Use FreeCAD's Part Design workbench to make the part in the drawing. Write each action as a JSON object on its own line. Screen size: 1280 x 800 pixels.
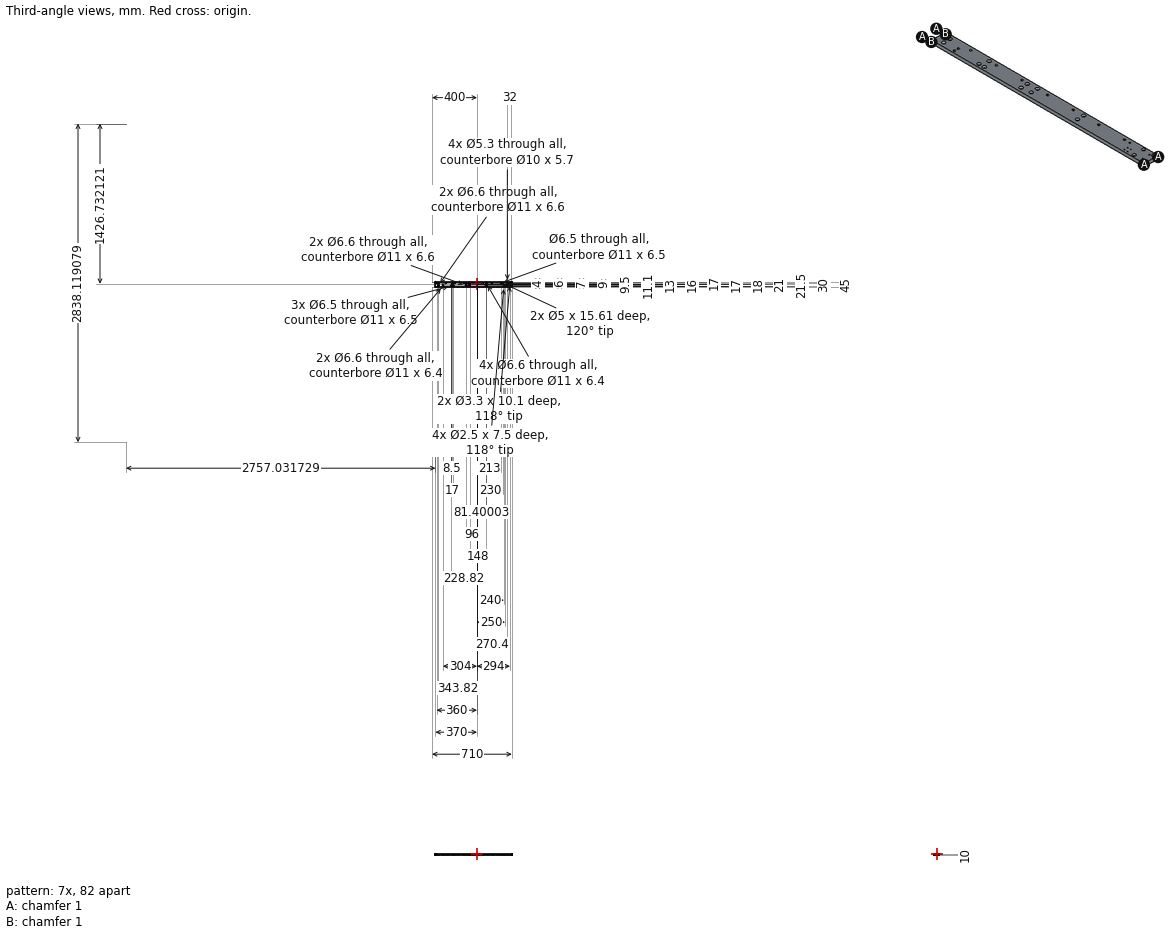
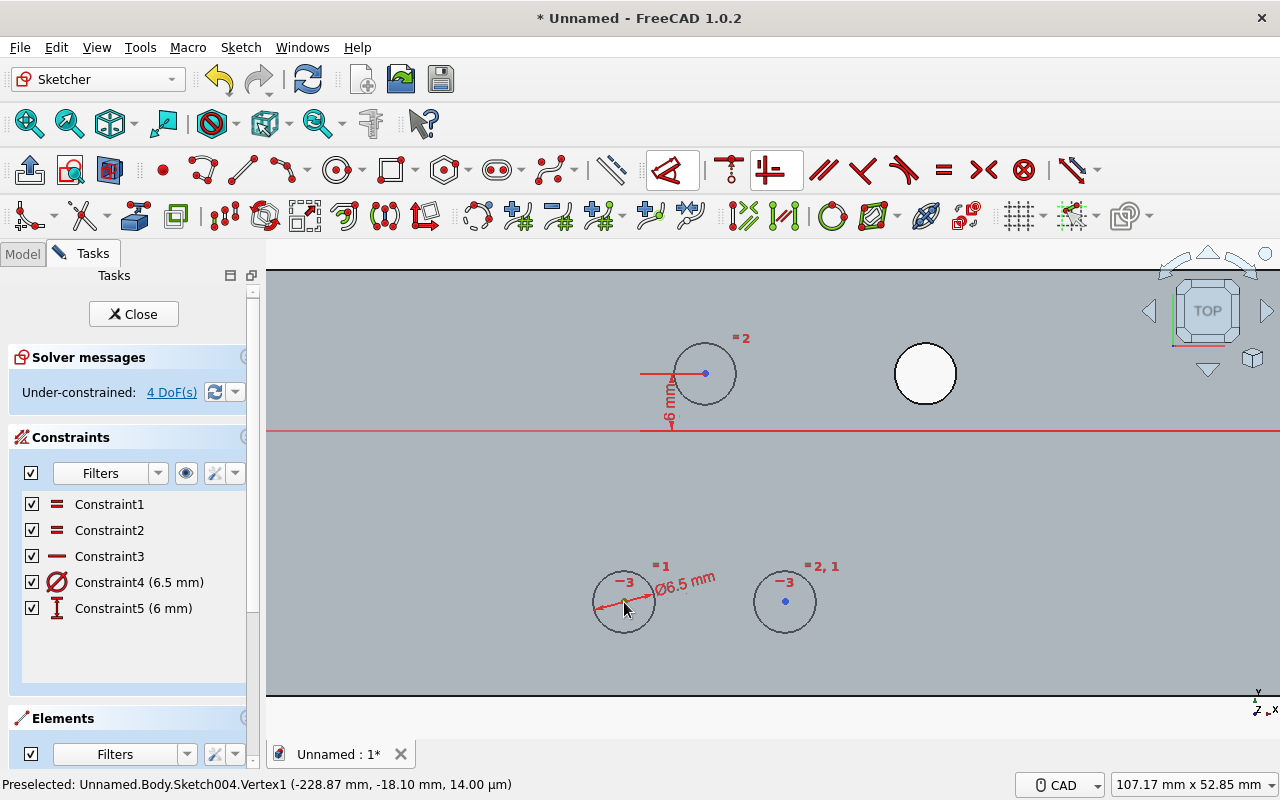
{"action": "left_click", "coordinate": [694, 170]}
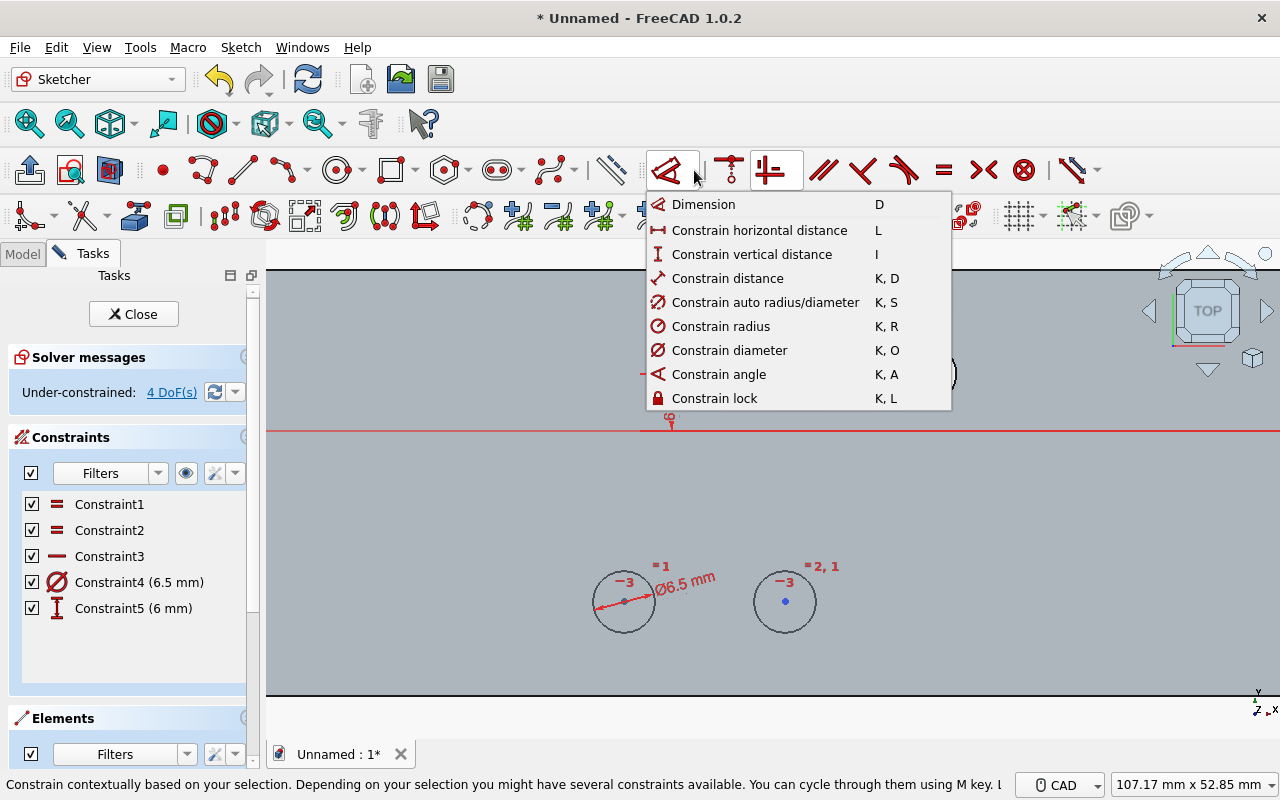
{"action": "left_click", "coordinate": [799, 254]}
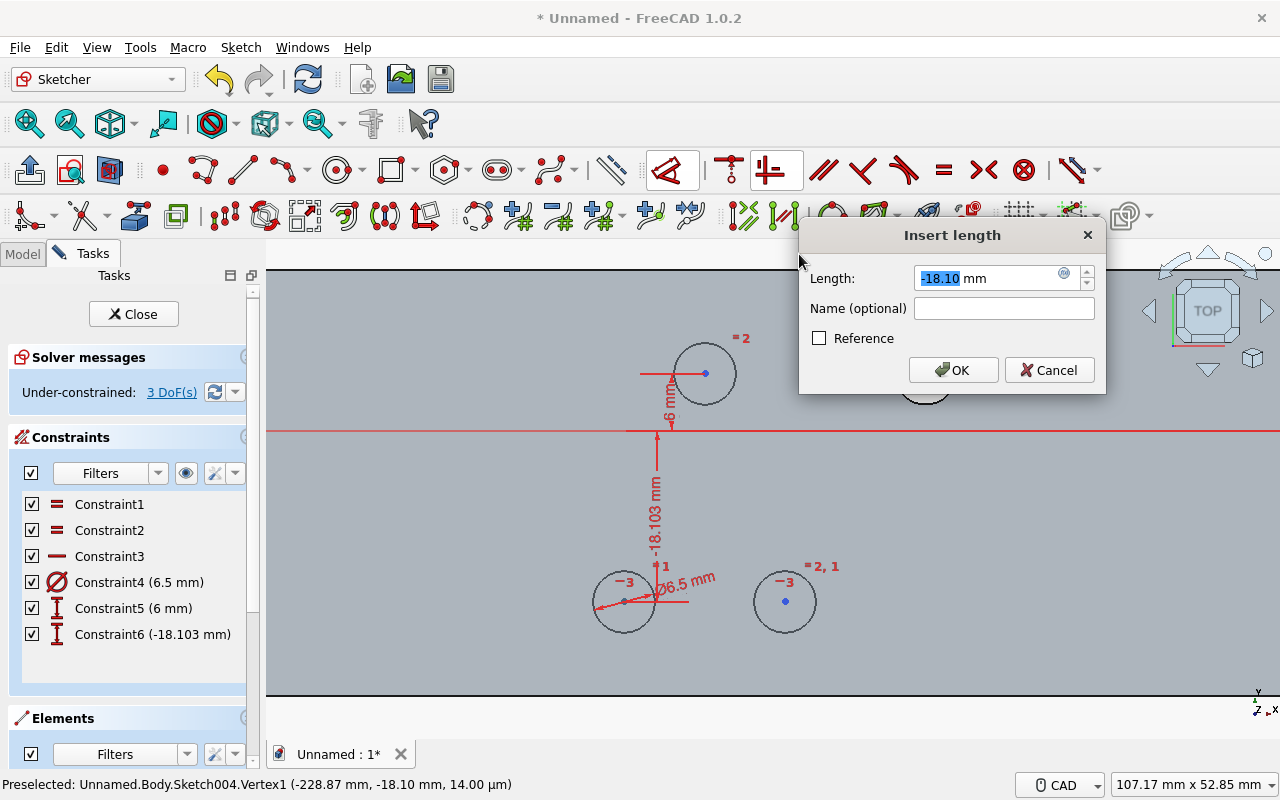
{"action": "type", "text": "-18"}
{"action": "key", "text": "Return"}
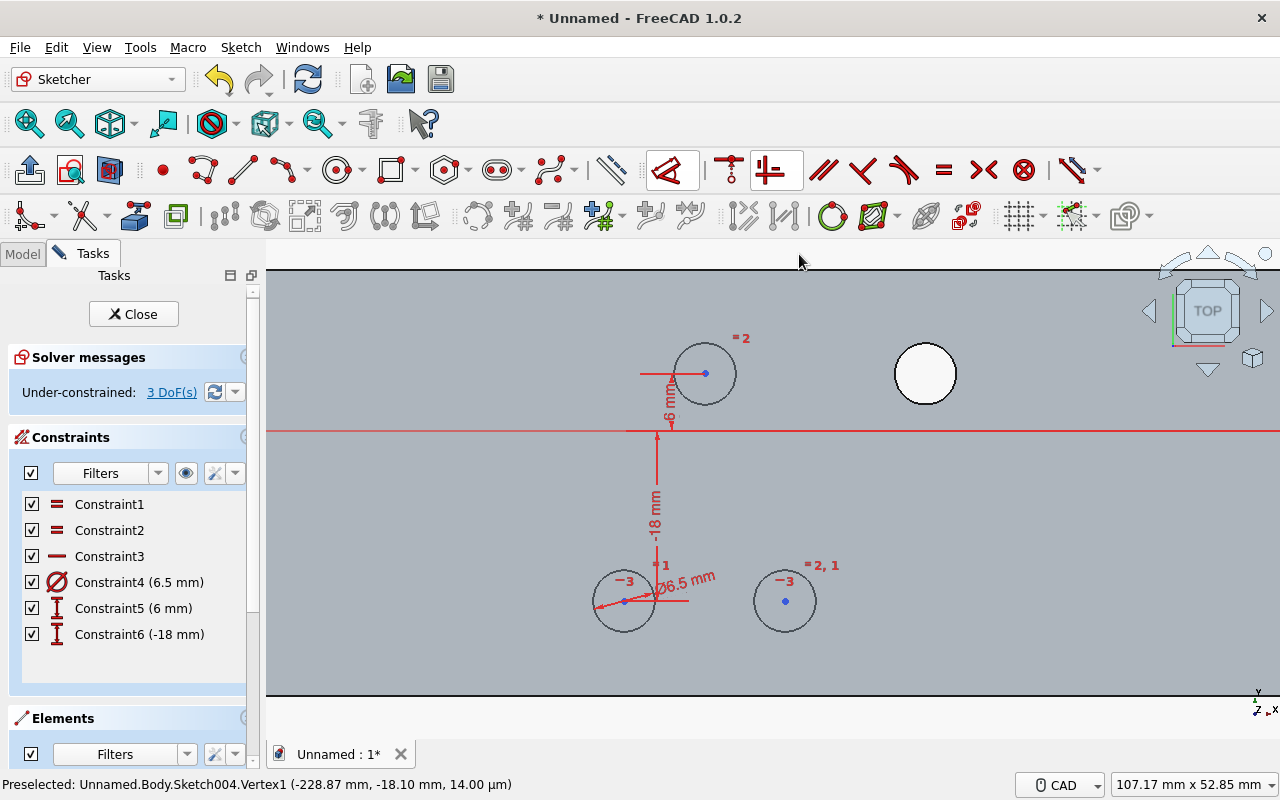
{"action": "left_click", "coordinate": [624, 601]}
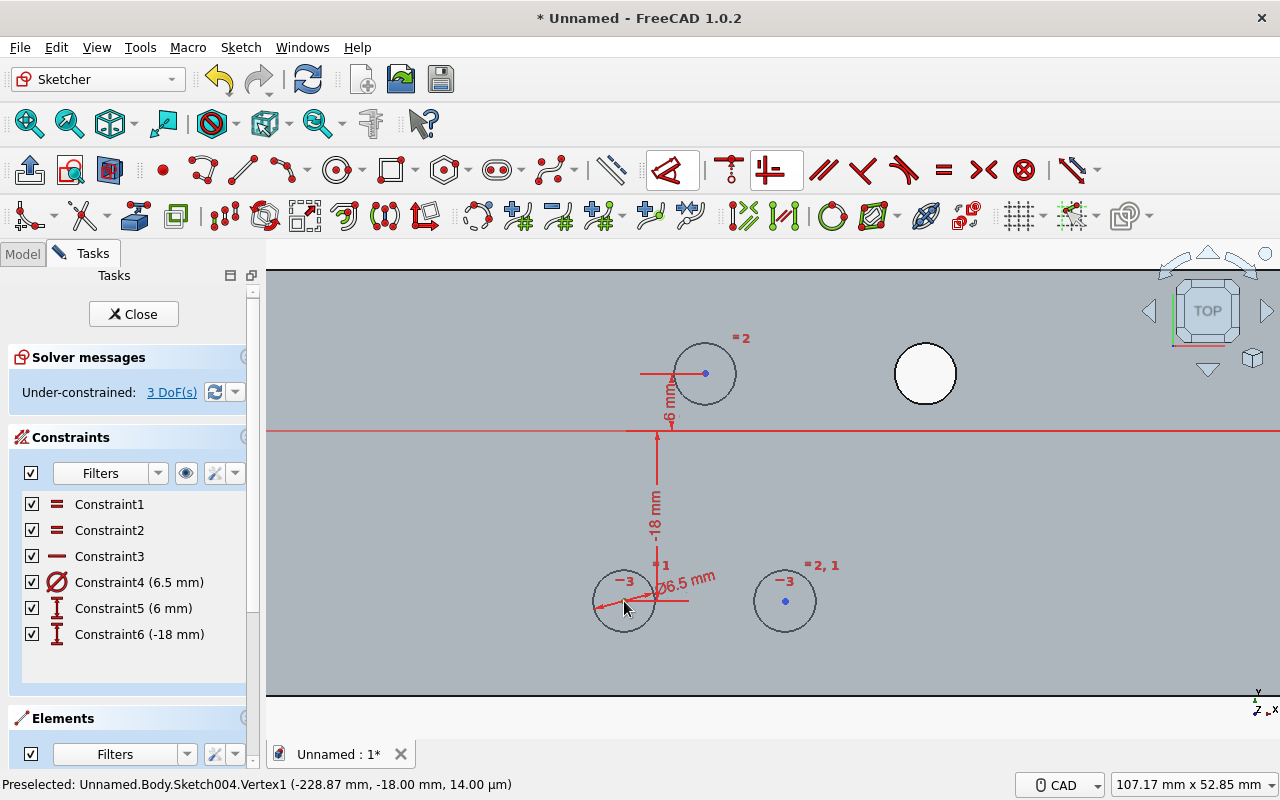
{"action": "left_click", "coordinate": [785, 601]}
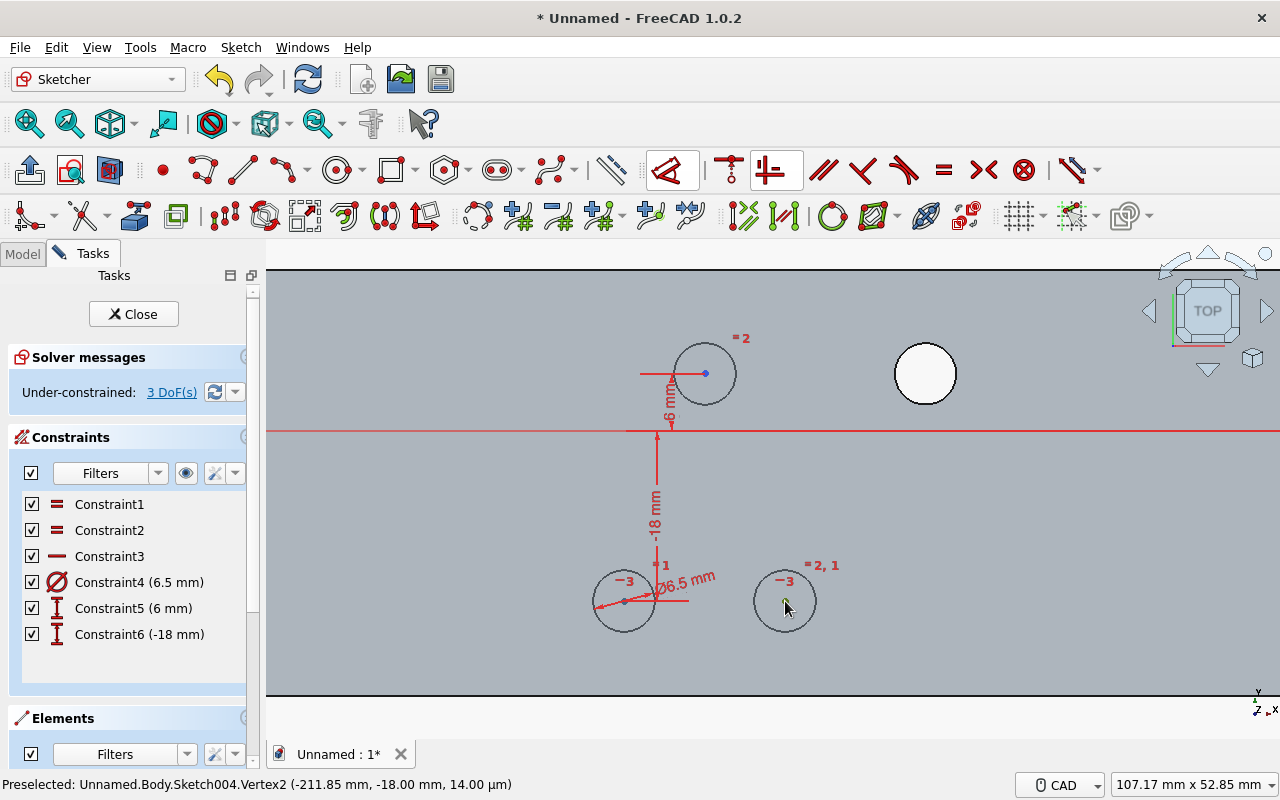
{"action": "left_click", "coordinate": [694, 170]}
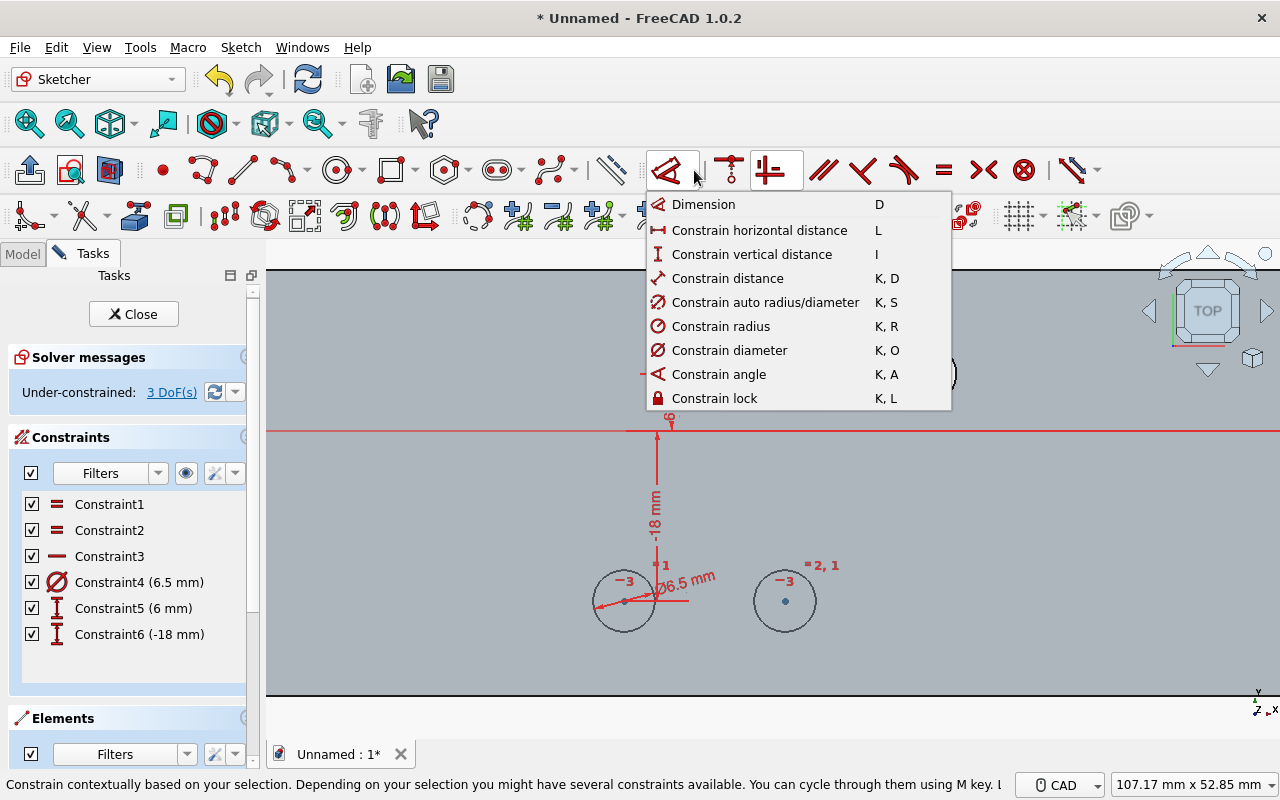
{"action": "left_click", "coordinate": [799, 230]}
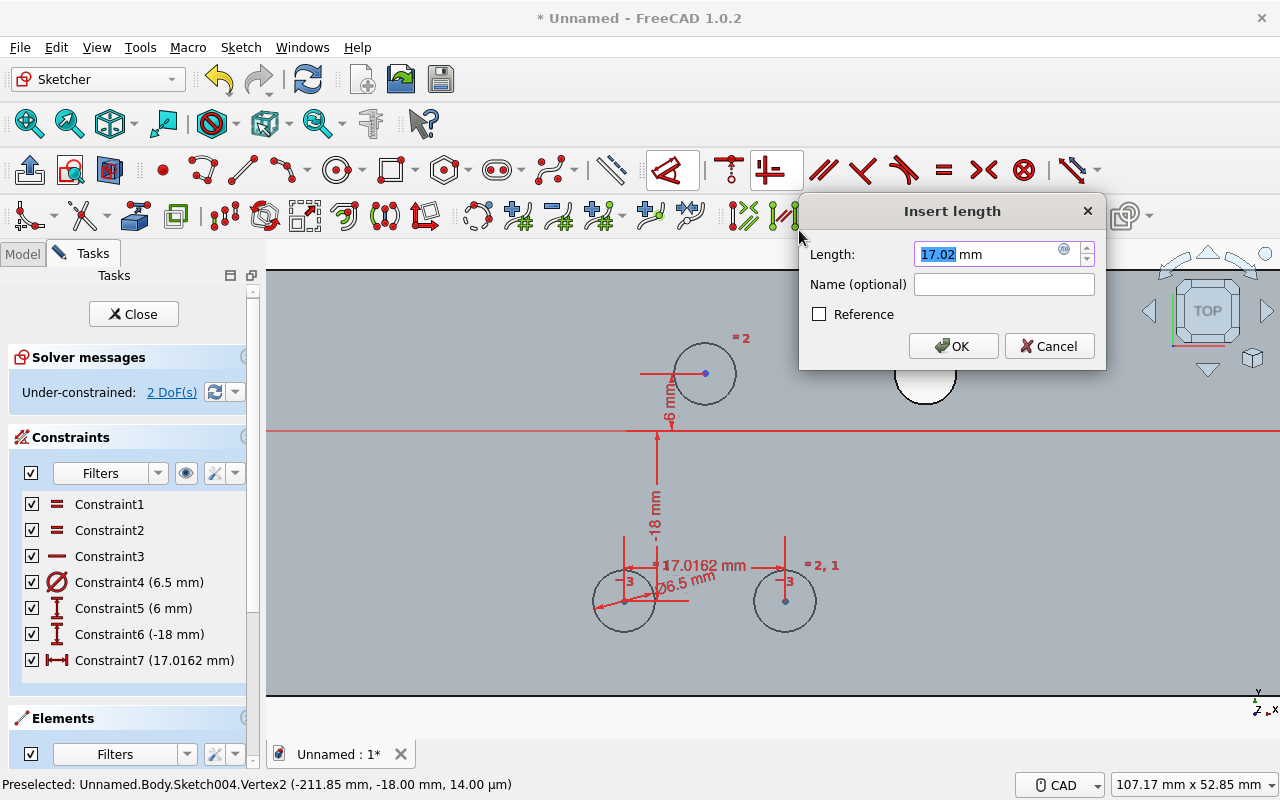
{"action": "type", "text": "17"}
{"action": "key", "text": "Return"}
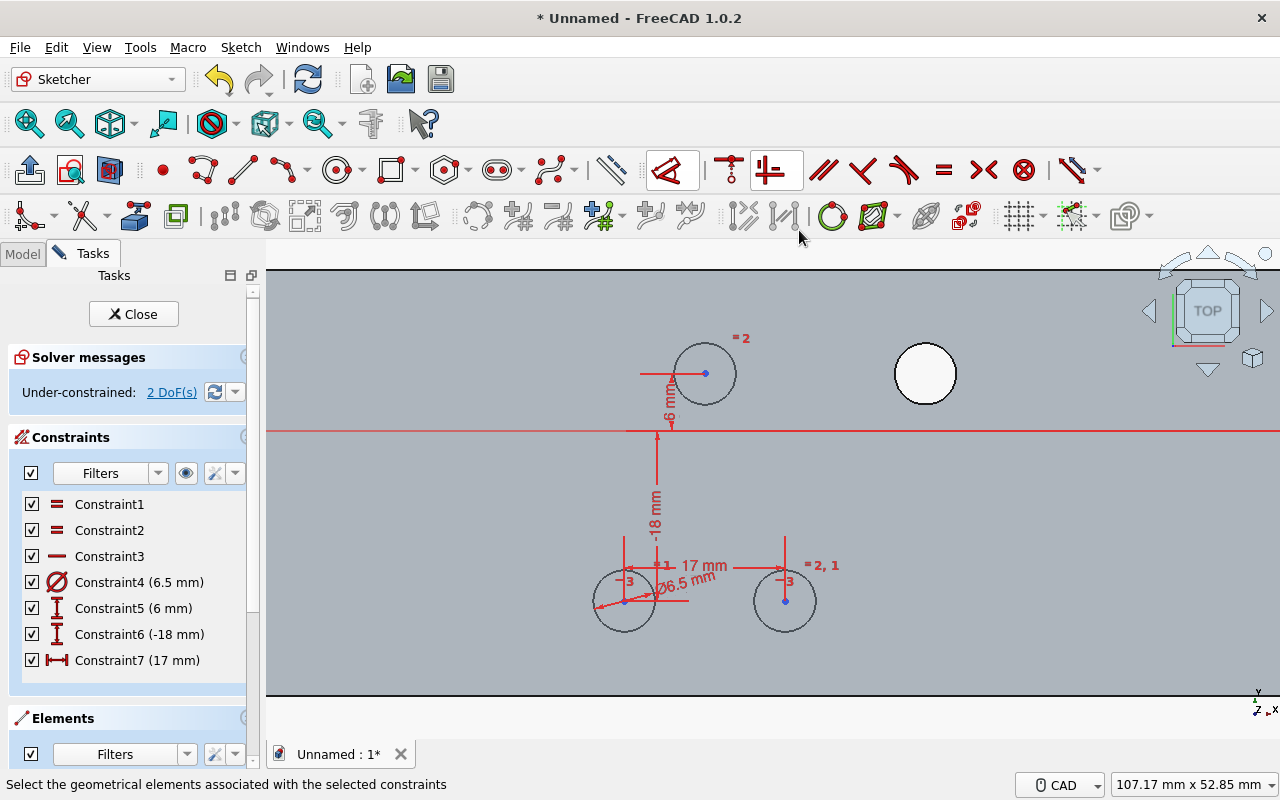
{"action": "left_click", "coordinate": [624, 601]}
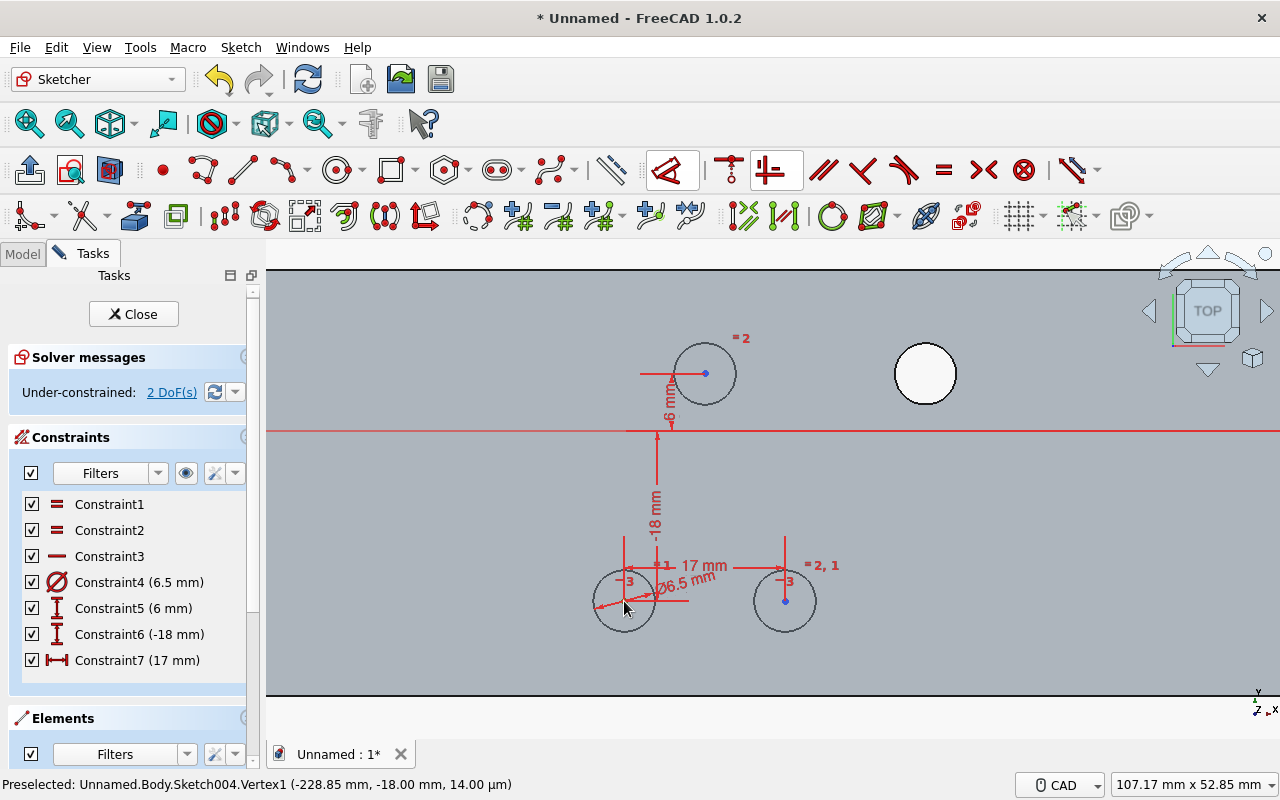
{"action": "left_click", "coordinate": [705, 374]}